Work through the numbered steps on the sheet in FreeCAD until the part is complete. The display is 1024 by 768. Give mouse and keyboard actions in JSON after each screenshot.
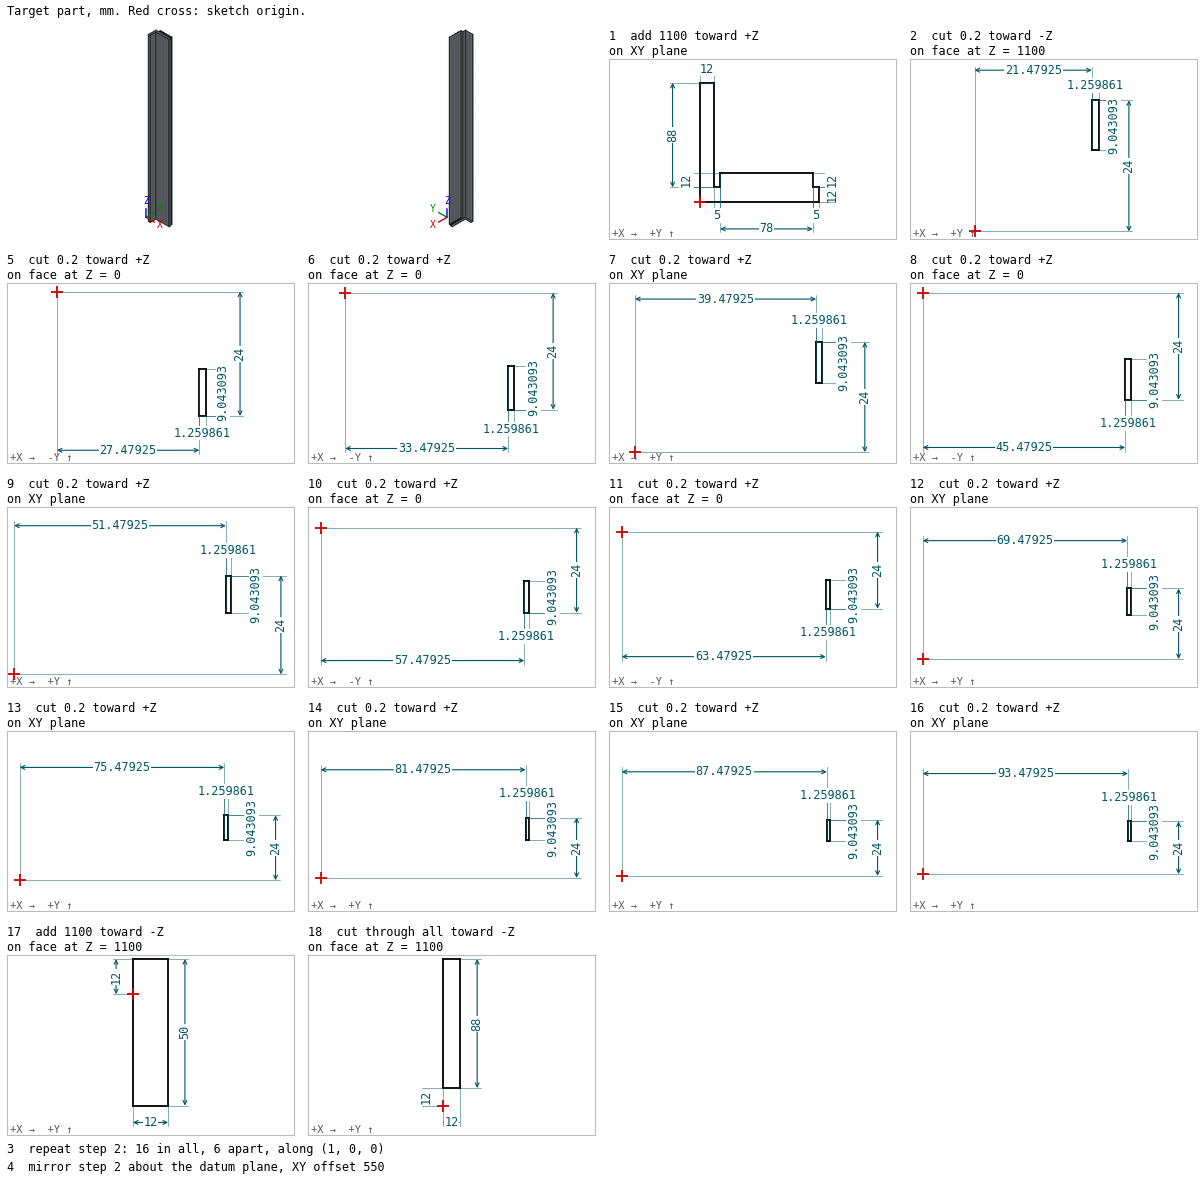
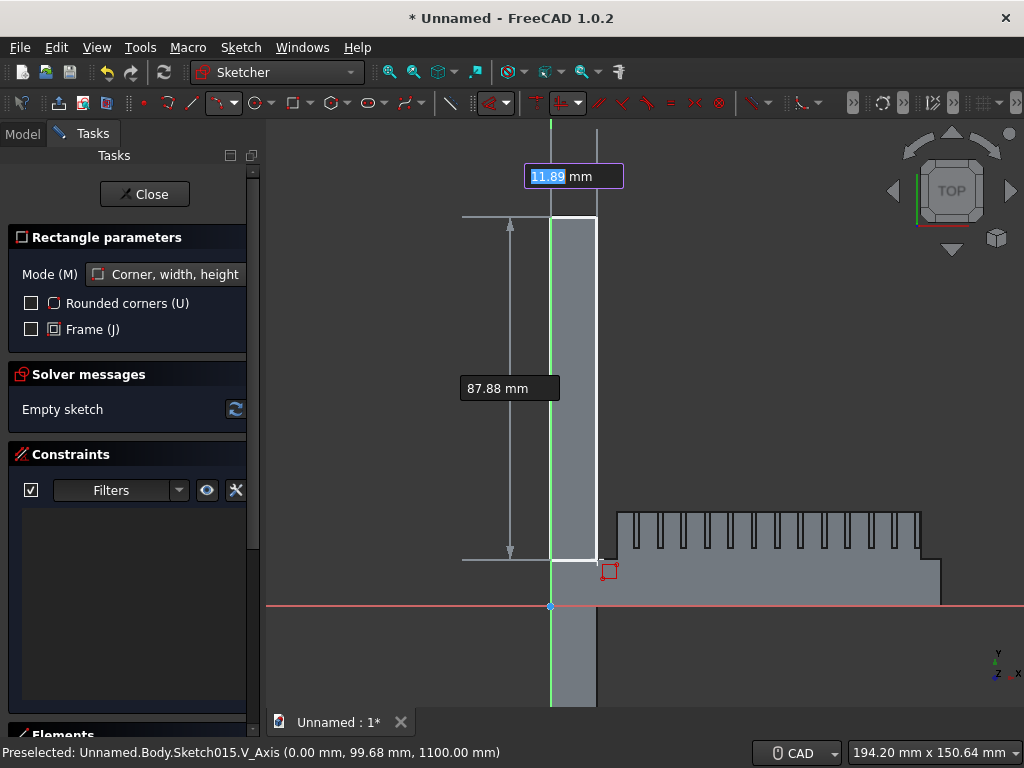
{"action": "type", "text": "12"}
{"action": "key", "text": "Tab"}
{"action": "type", "text": "88"}
{"action": "key", "text": "Return"}
{"action": "key", "text": "Escape"}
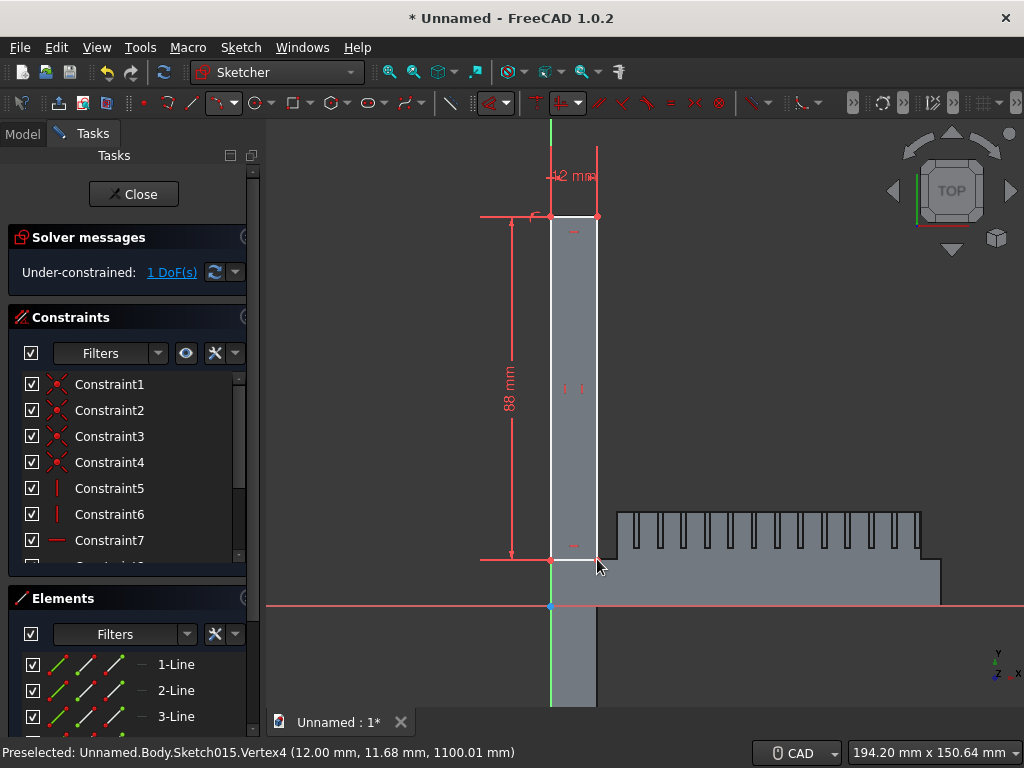
{"action": "left_click", "coordinate": [551, 560]}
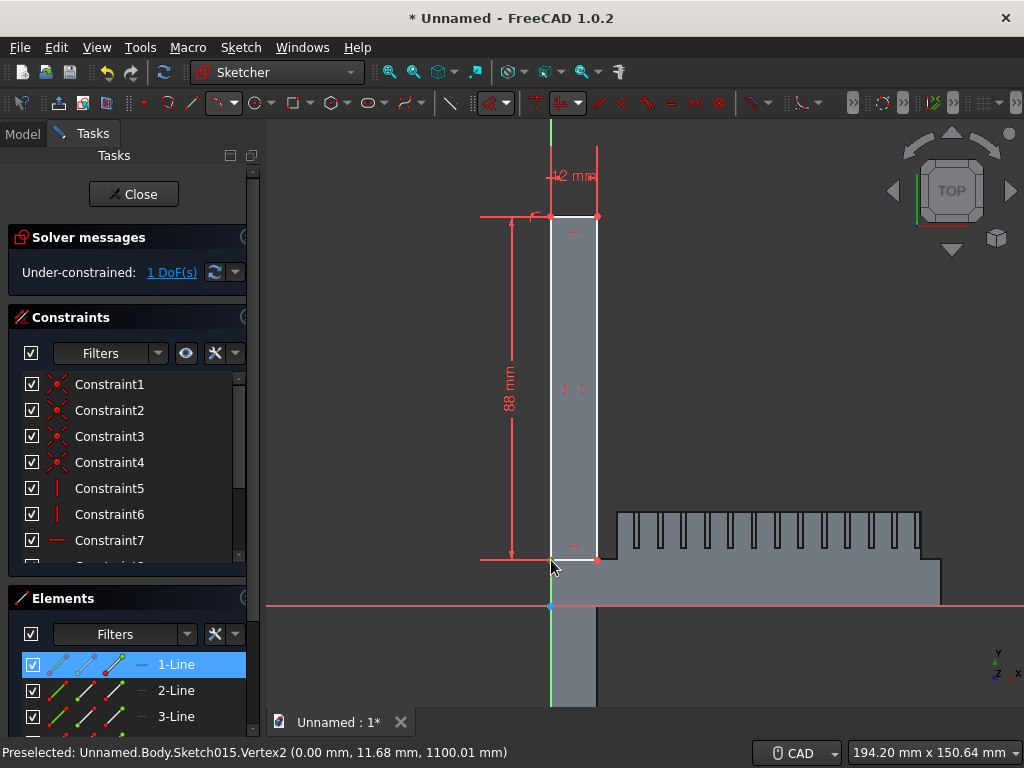
{"action": "key", "text": "i"}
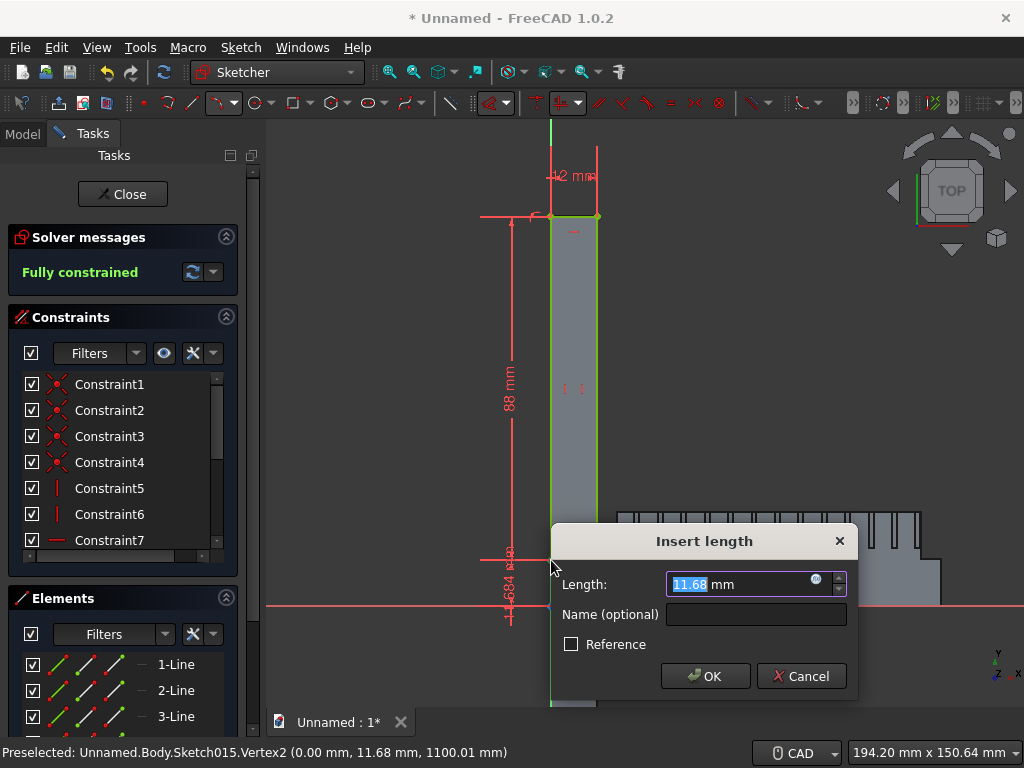
{"action": "type", "text": "12"}
{"action": "key", "text": "Return"}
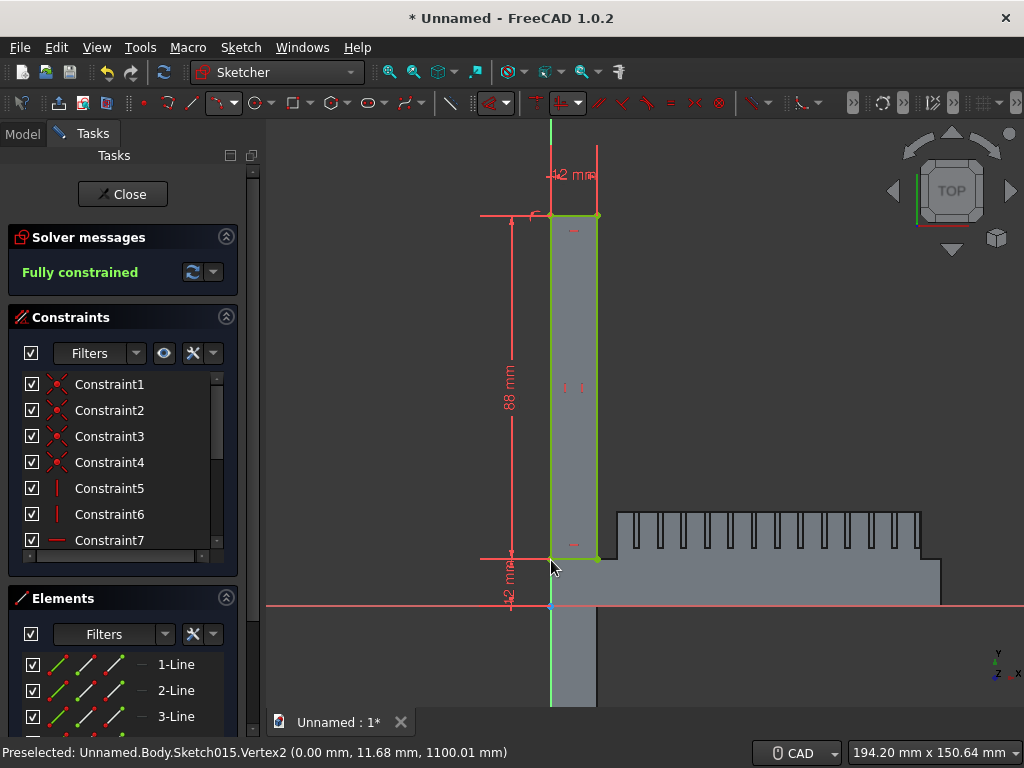
{"action": "left_click", "coordinate": [123, 194]}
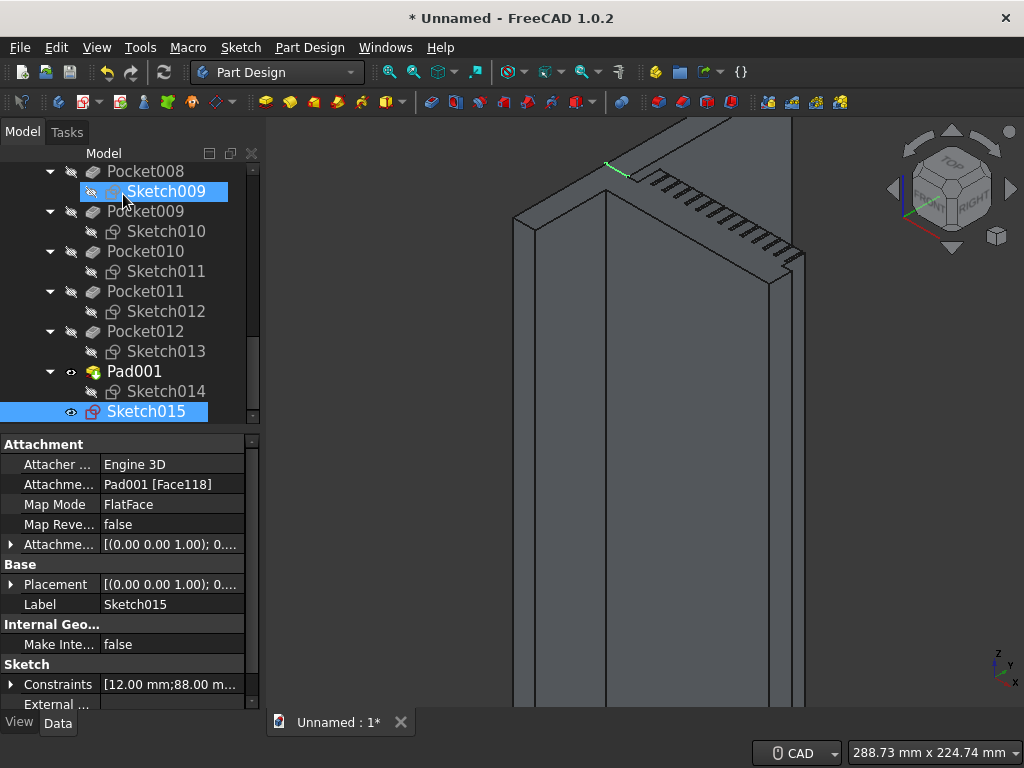
{"action": "left_click", "coordinate": [432, 102]}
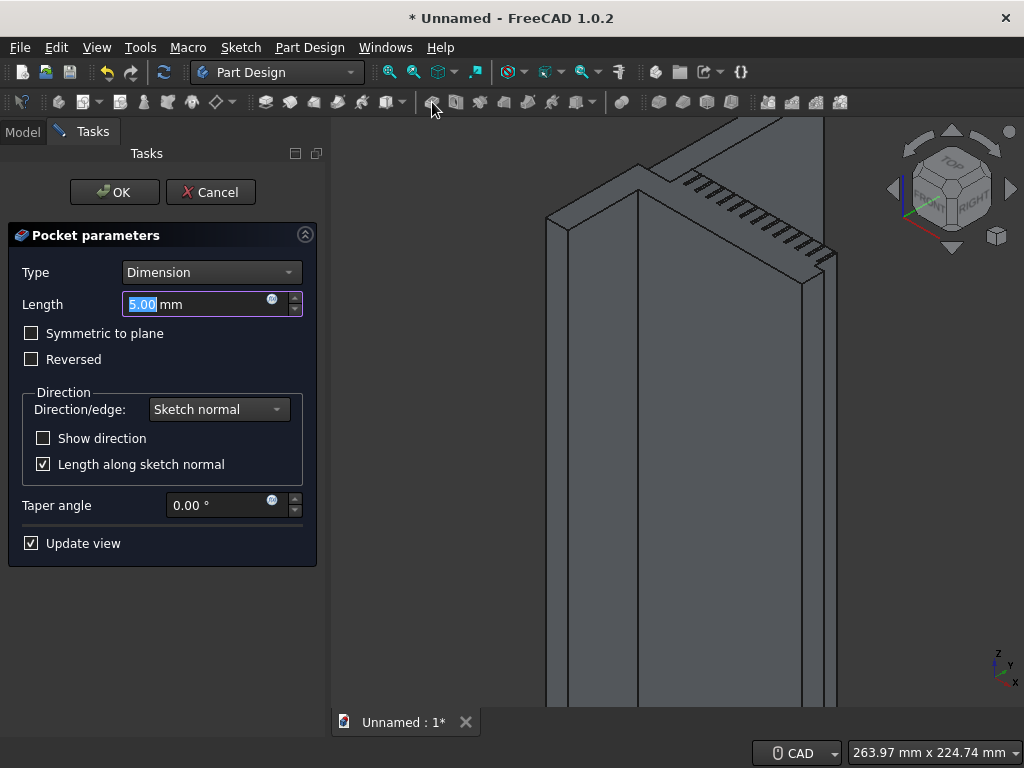
{"action": "left_click", "coordinate": [212, 272]}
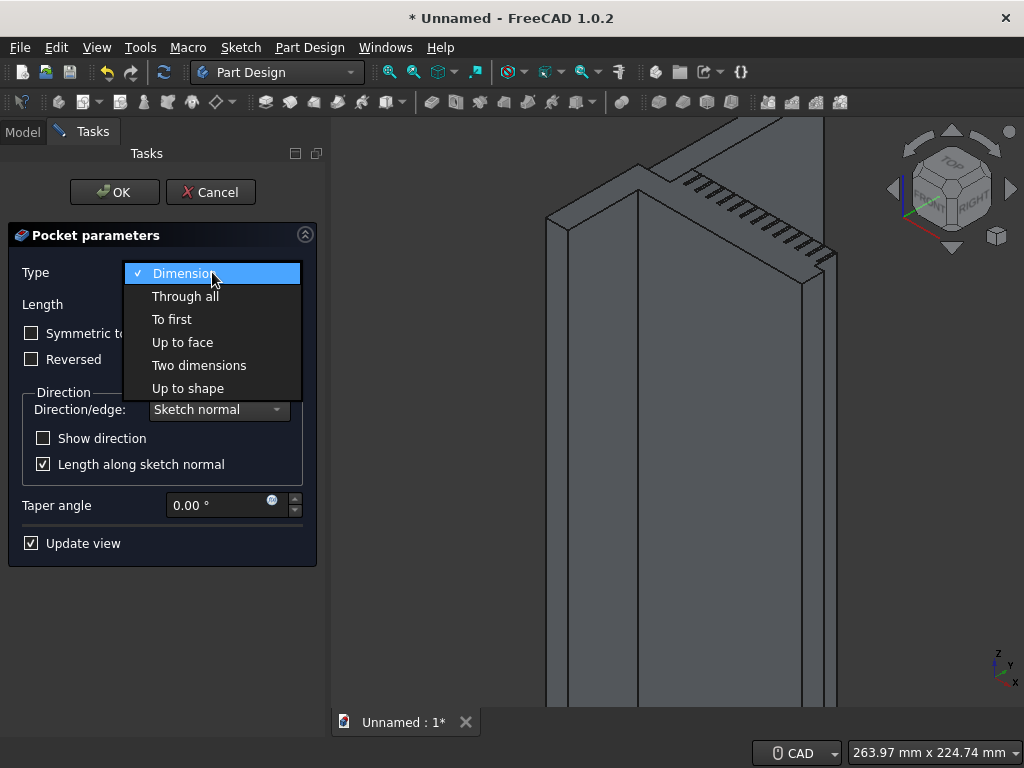
{"action": "left_click", "coordinate": [212, 296]}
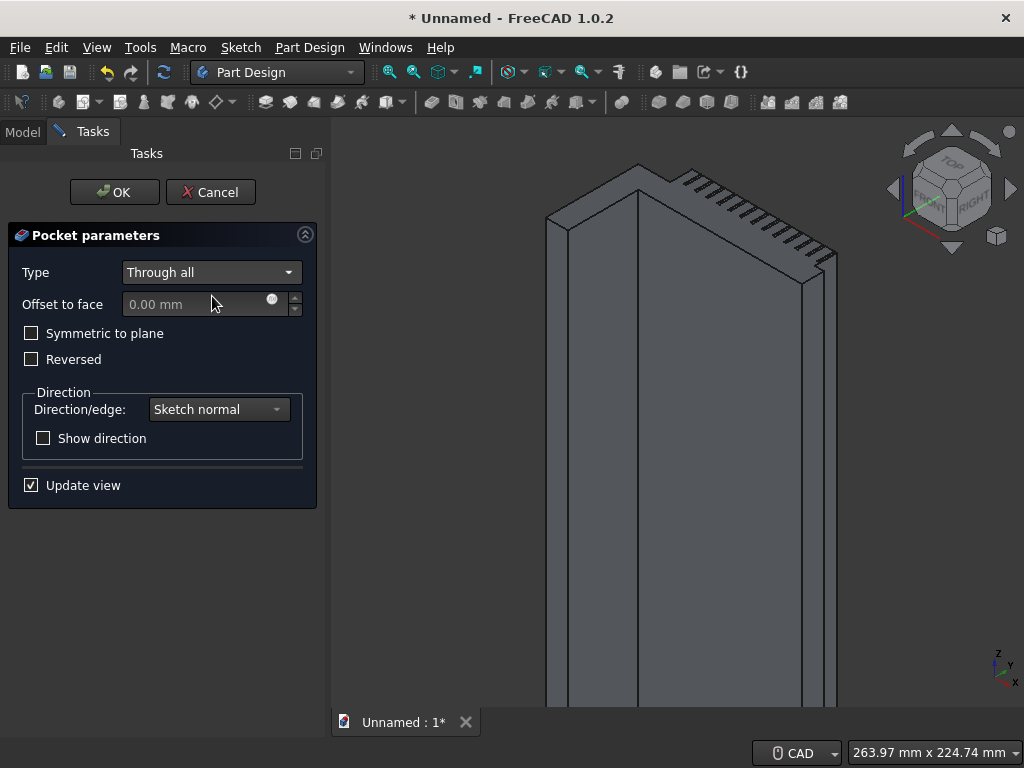
{"action": "left_click", "coordinate": [115, 192]}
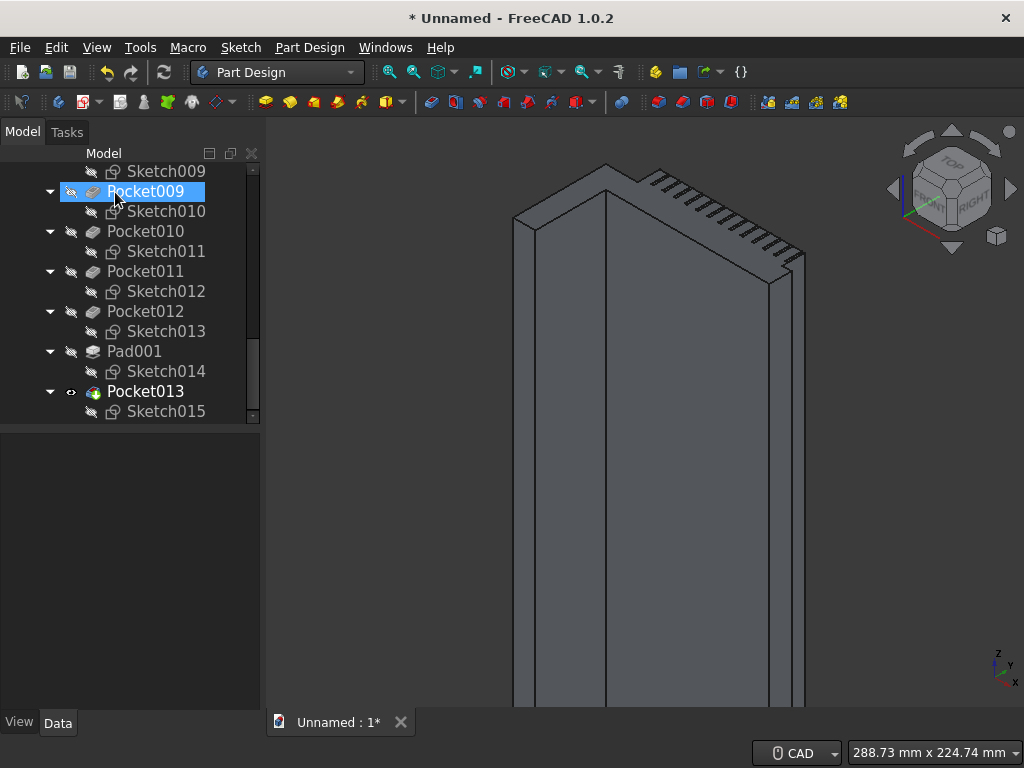
{"action": "left_click", "coordinate": [390, 72]}